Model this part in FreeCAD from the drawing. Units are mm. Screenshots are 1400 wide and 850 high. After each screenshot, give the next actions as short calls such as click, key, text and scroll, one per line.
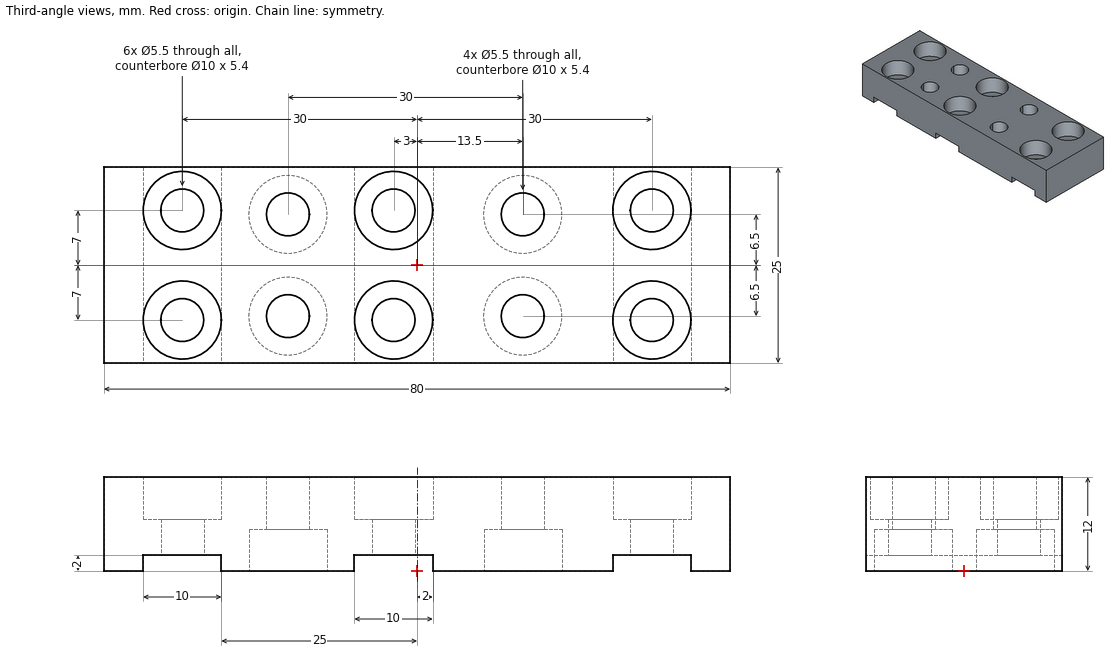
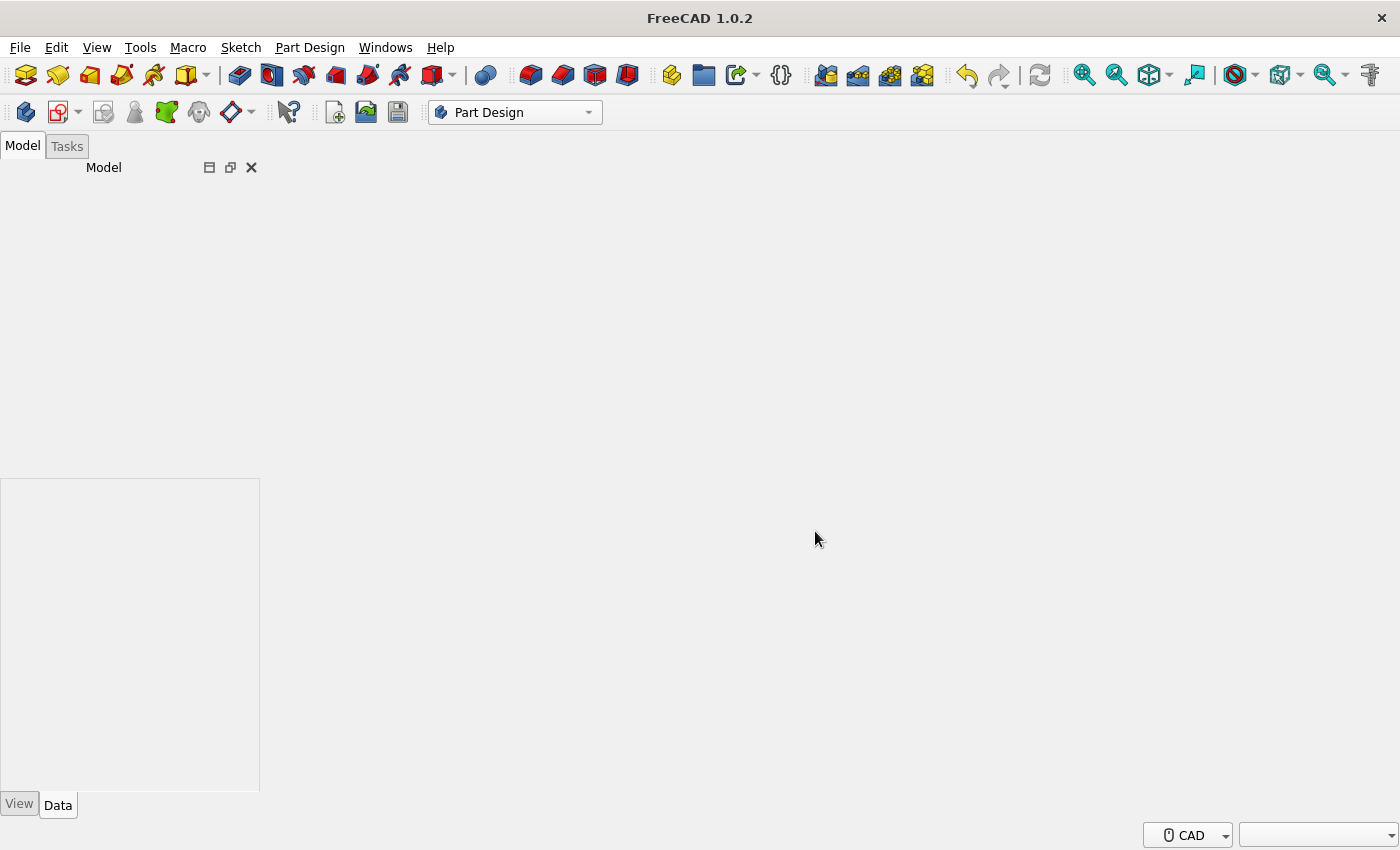
click(334, 112)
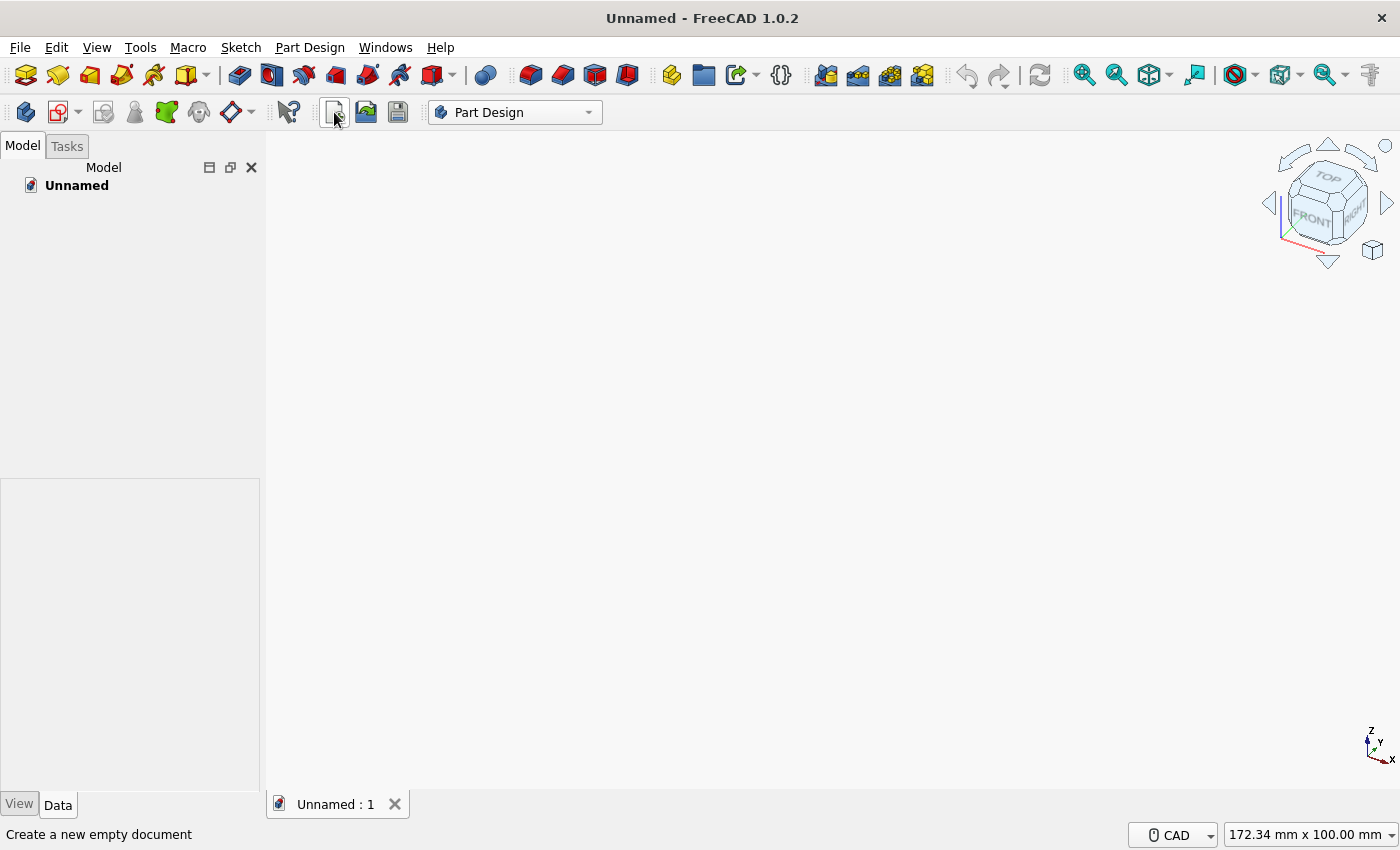
click(58, 112)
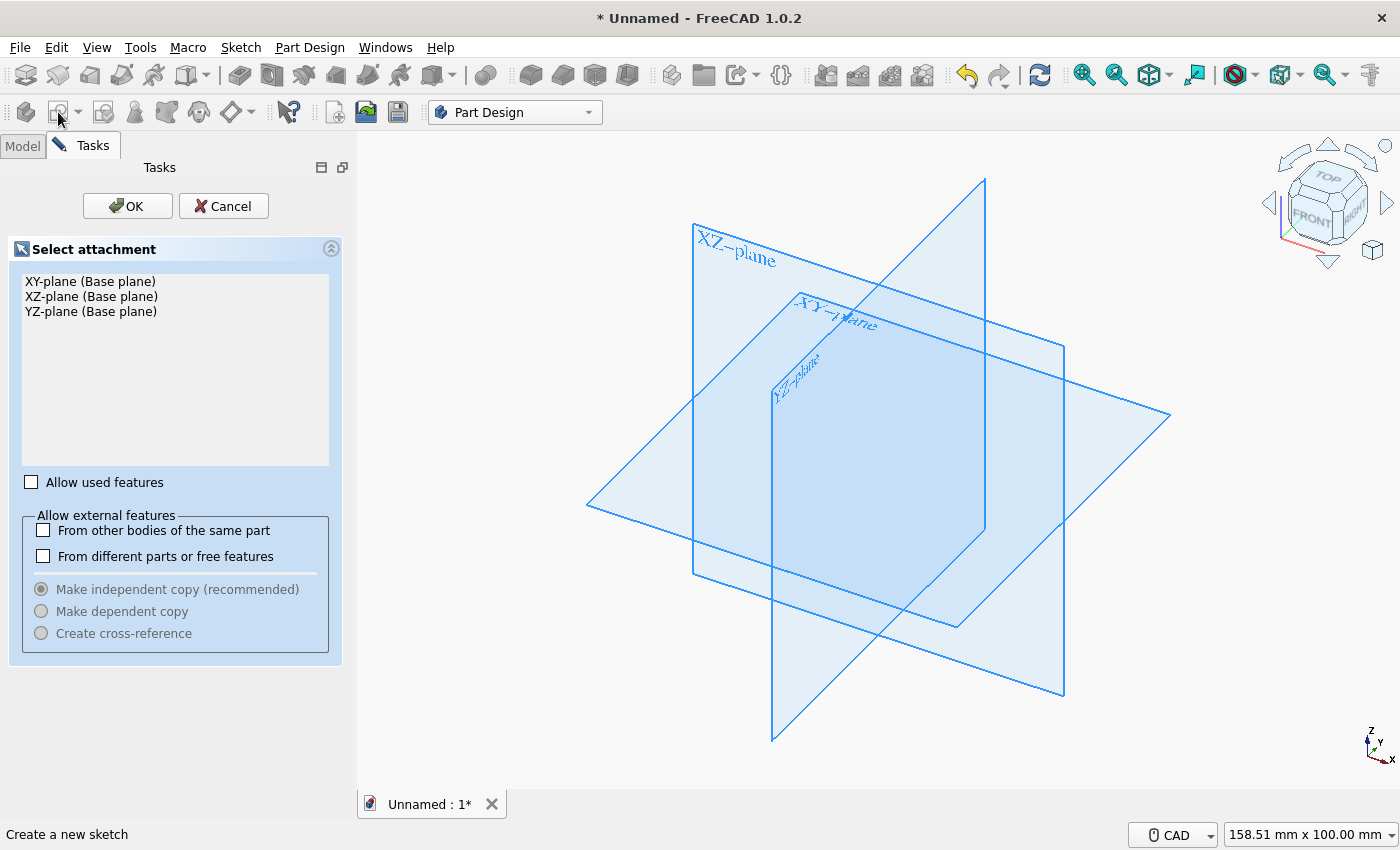
click(82, 282)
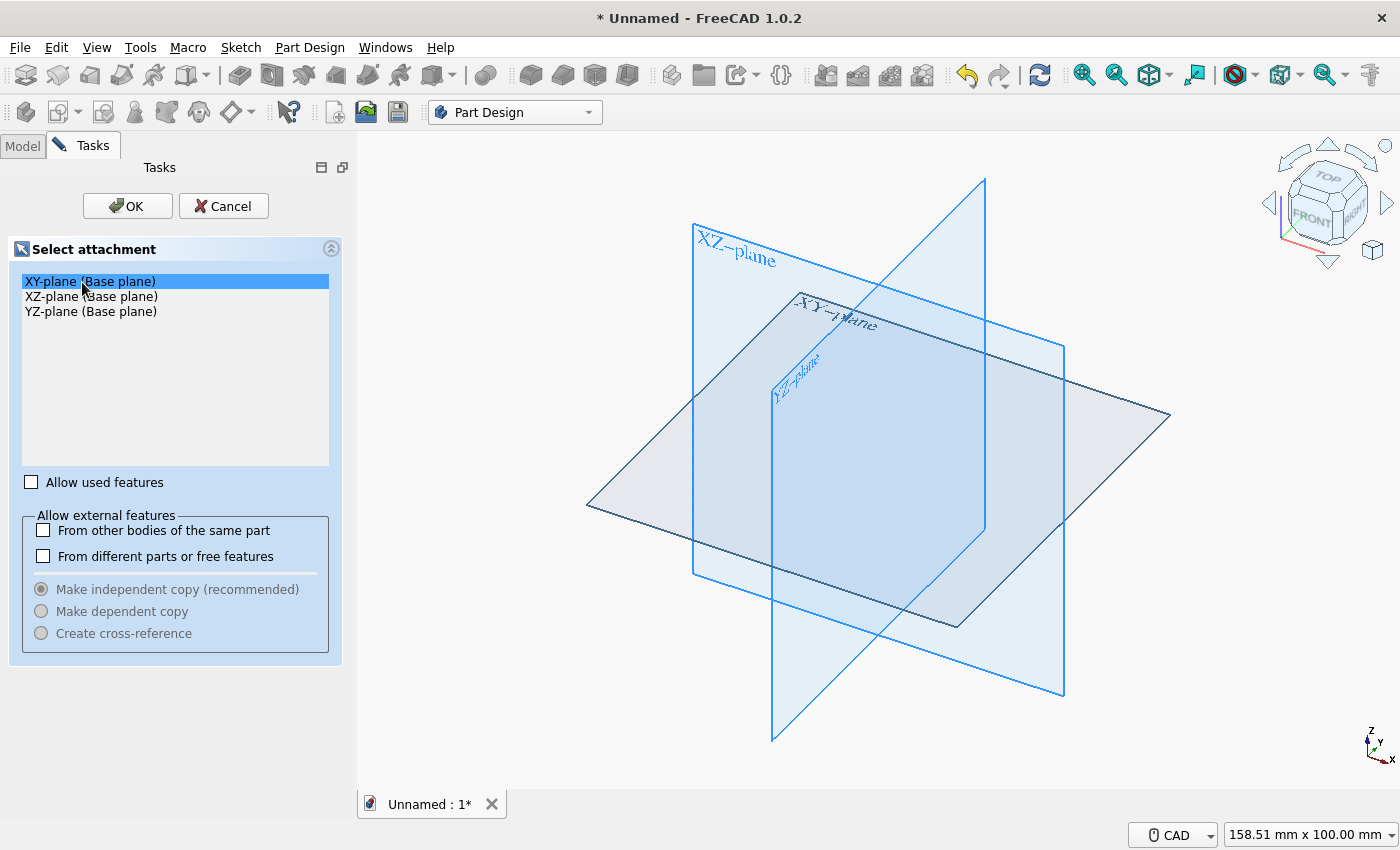
click(128, 206)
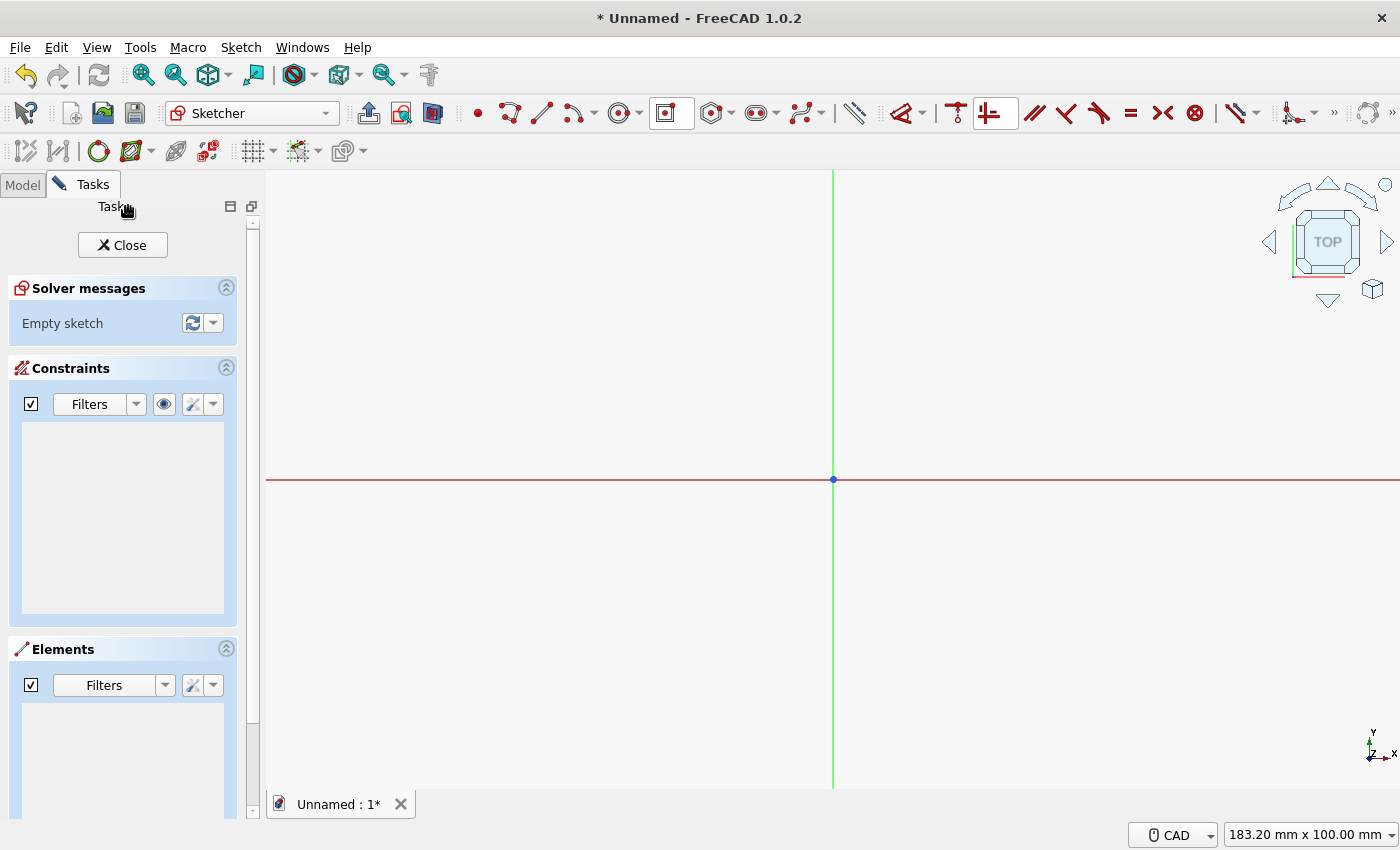
click(666, 114)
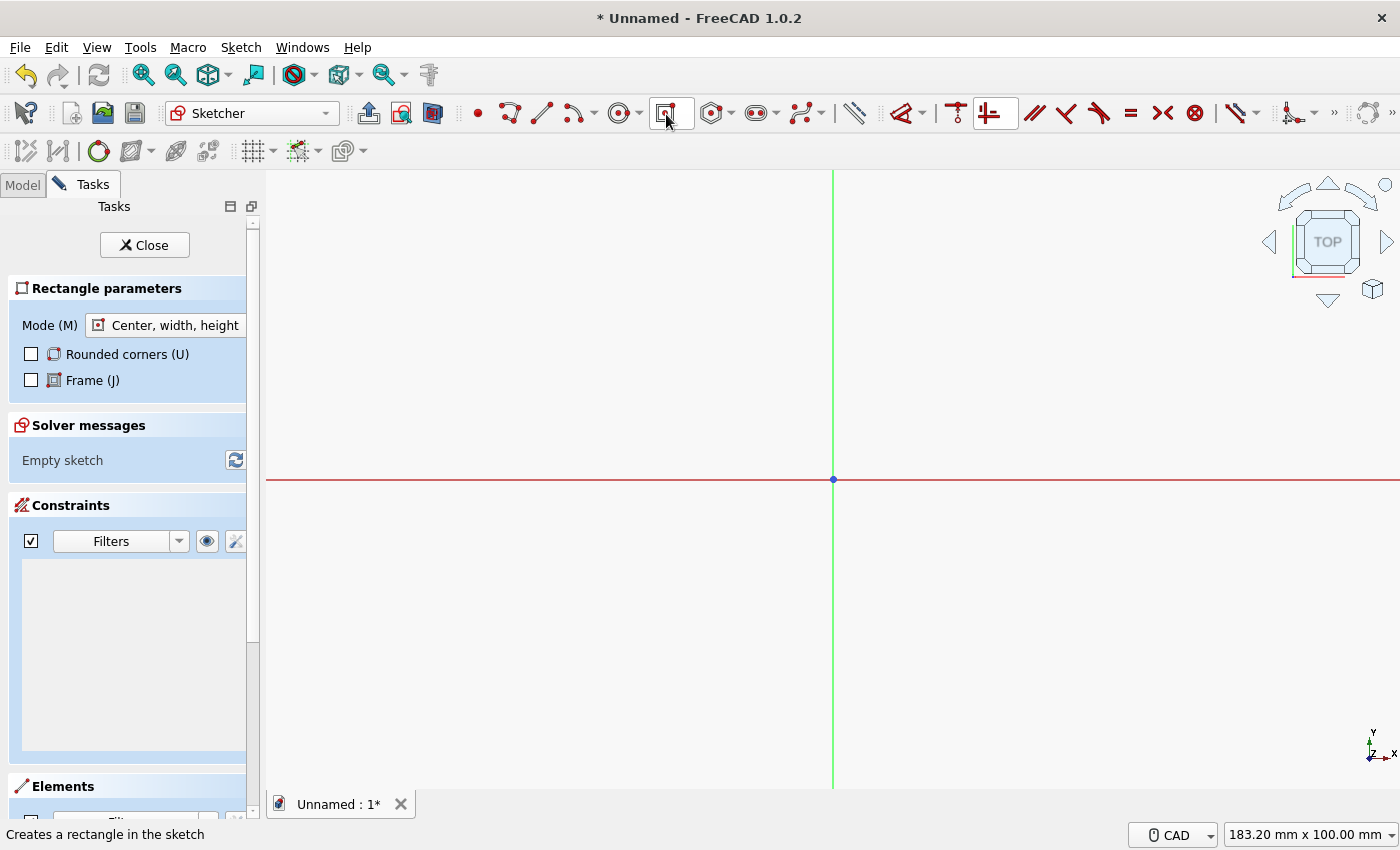
click(833, 480)
click(1081, 402)
key(Escape)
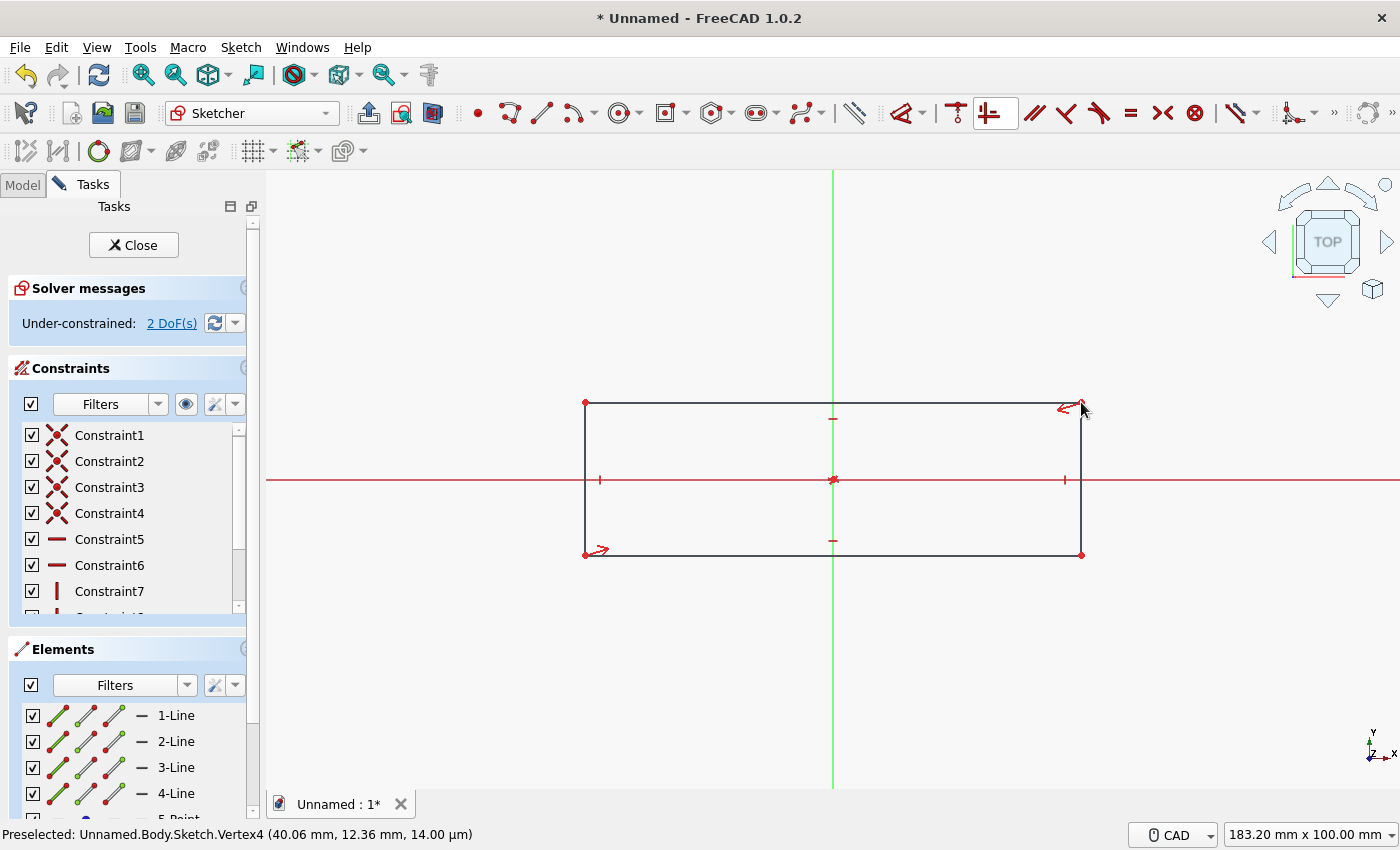
click(734, 556)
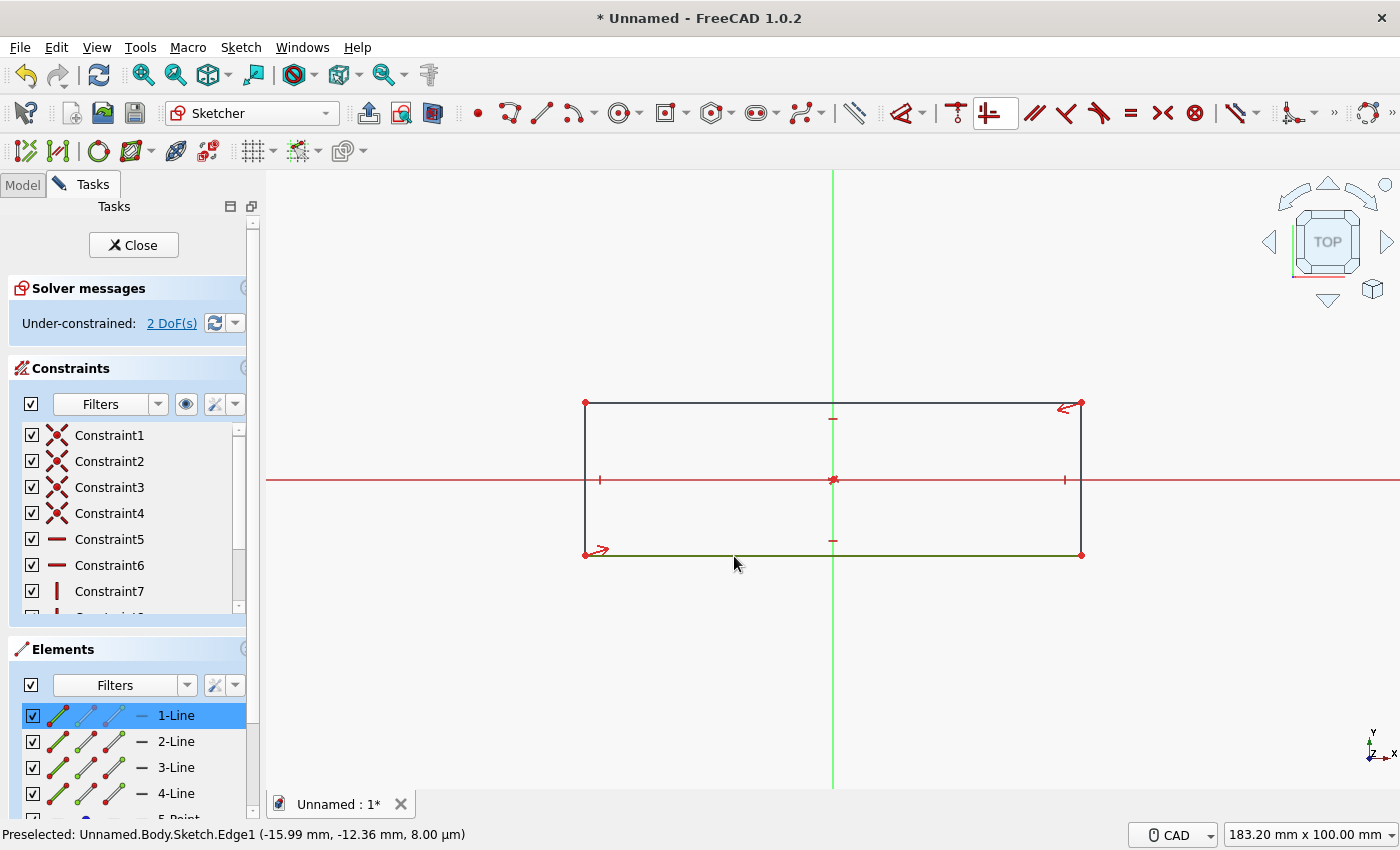
click(924, 114)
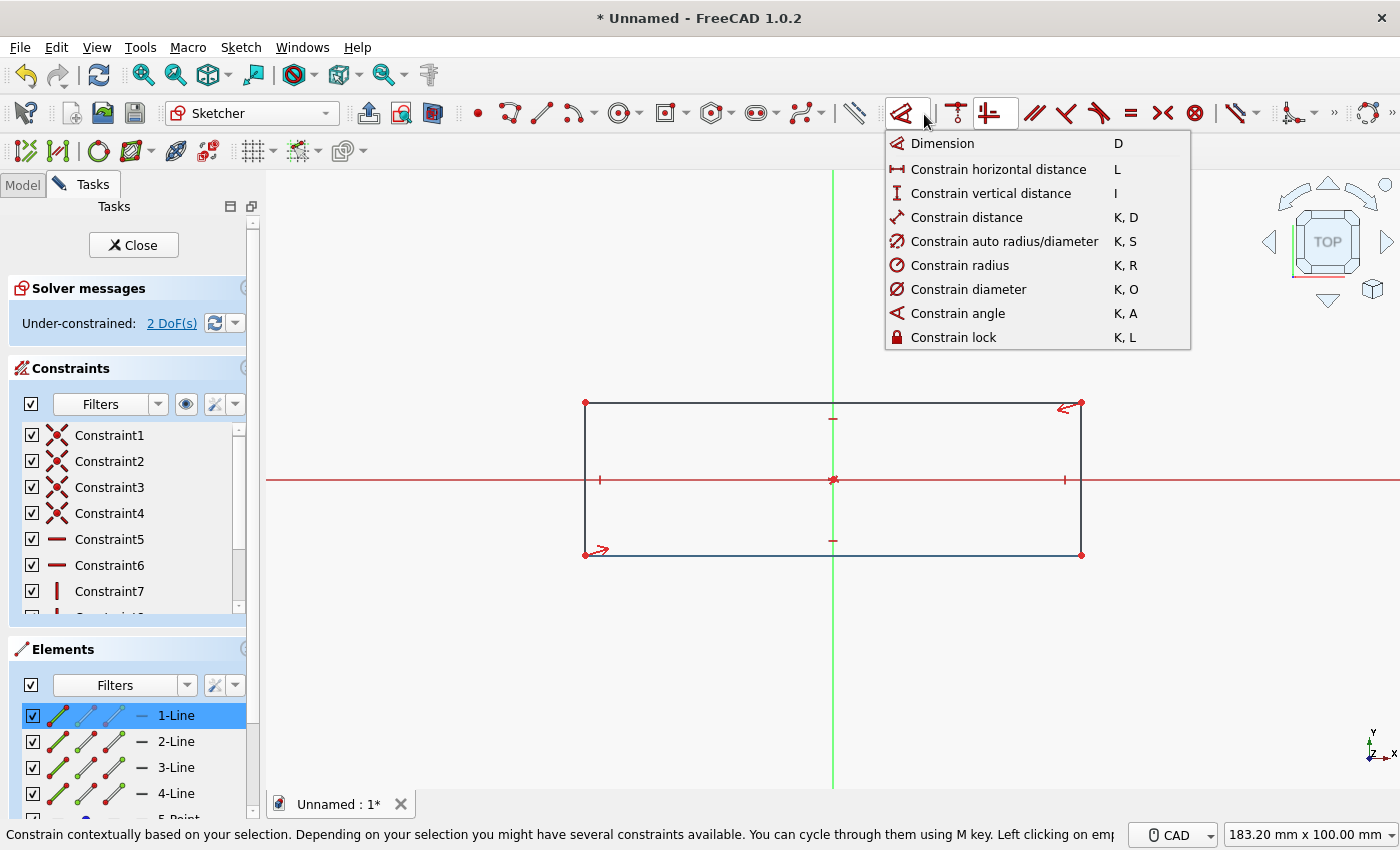
click(1038, 169)